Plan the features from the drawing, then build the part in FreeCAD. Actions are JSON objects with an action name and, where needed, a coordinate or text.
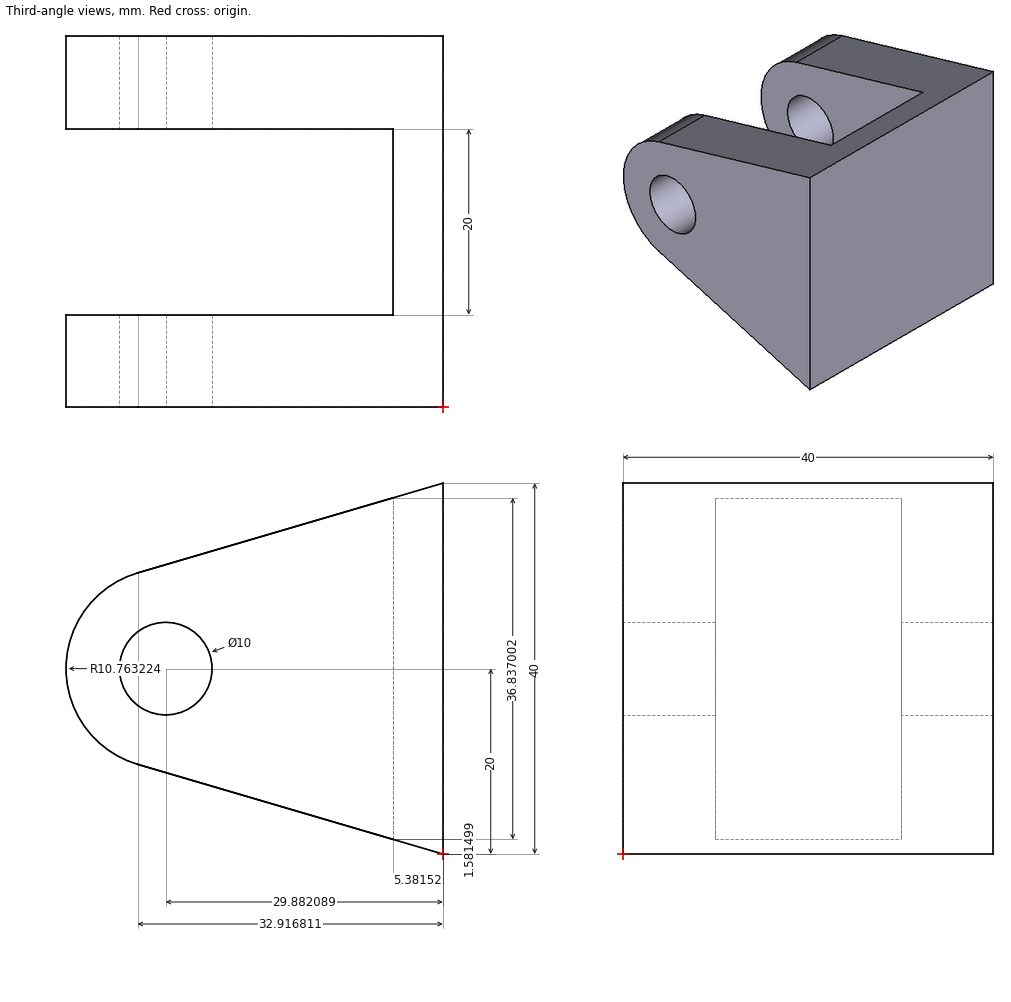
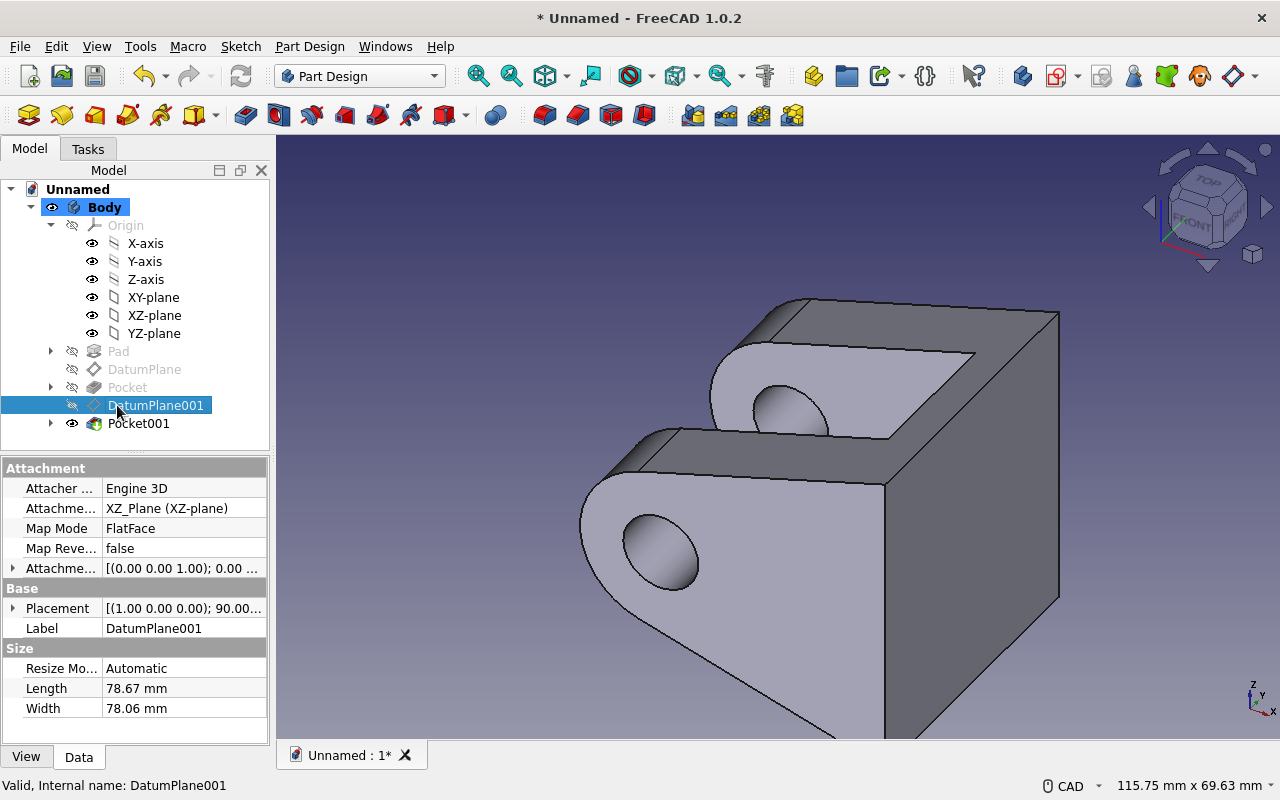
{"action": "key", "text": "0"}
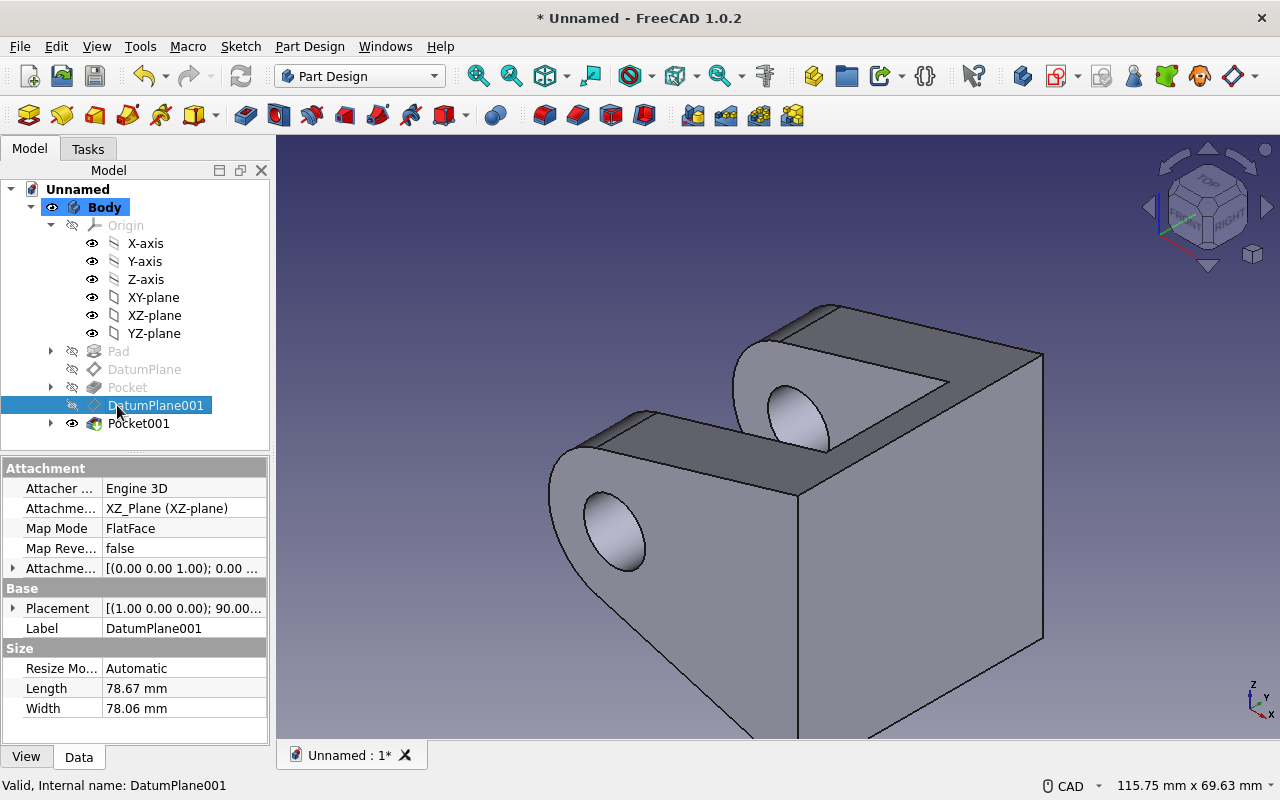
{"action": "left_click", "coordinate": [479, 76]}